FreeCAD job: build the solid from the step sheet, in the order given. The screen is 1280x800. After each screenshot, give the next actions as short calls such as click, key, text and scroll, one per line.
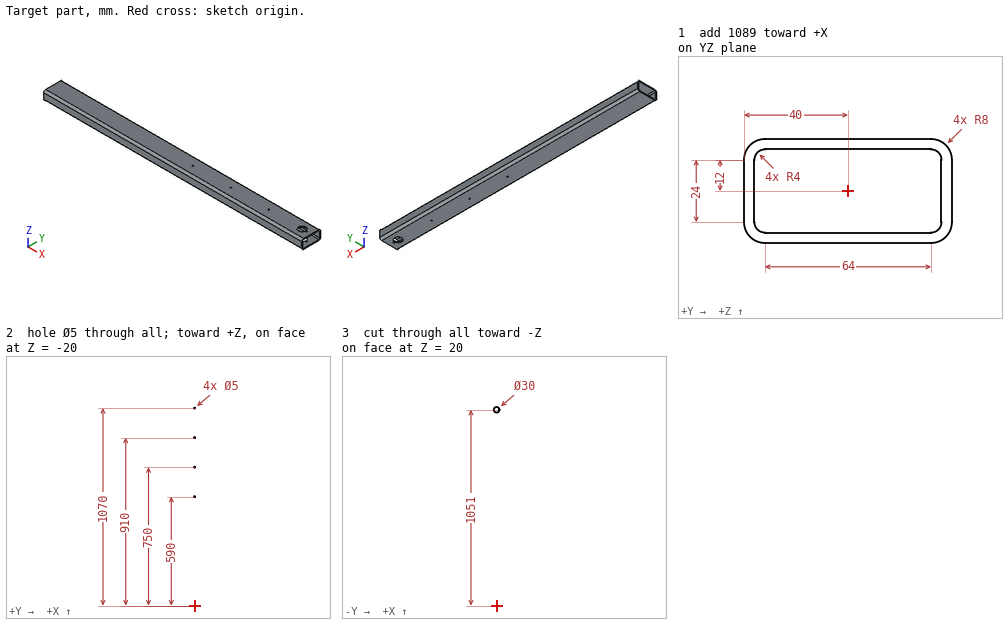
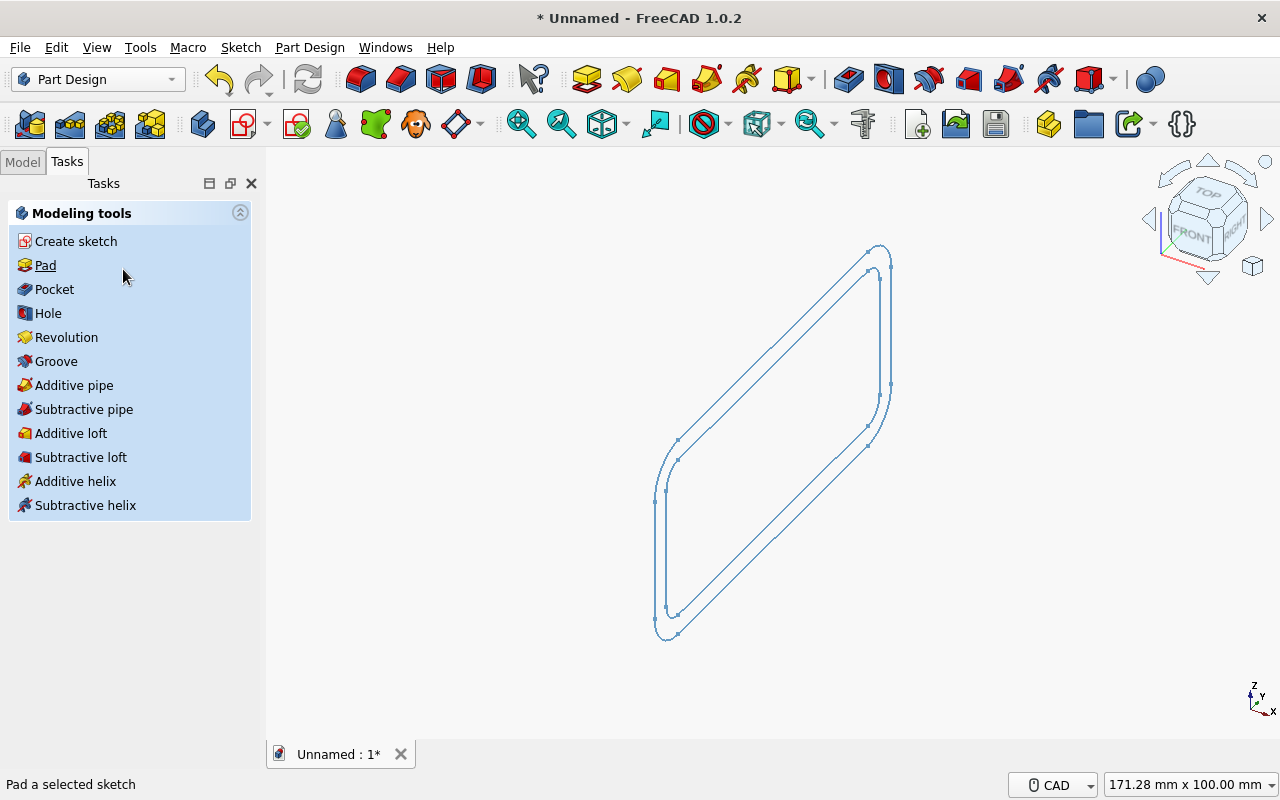
click(588, 80)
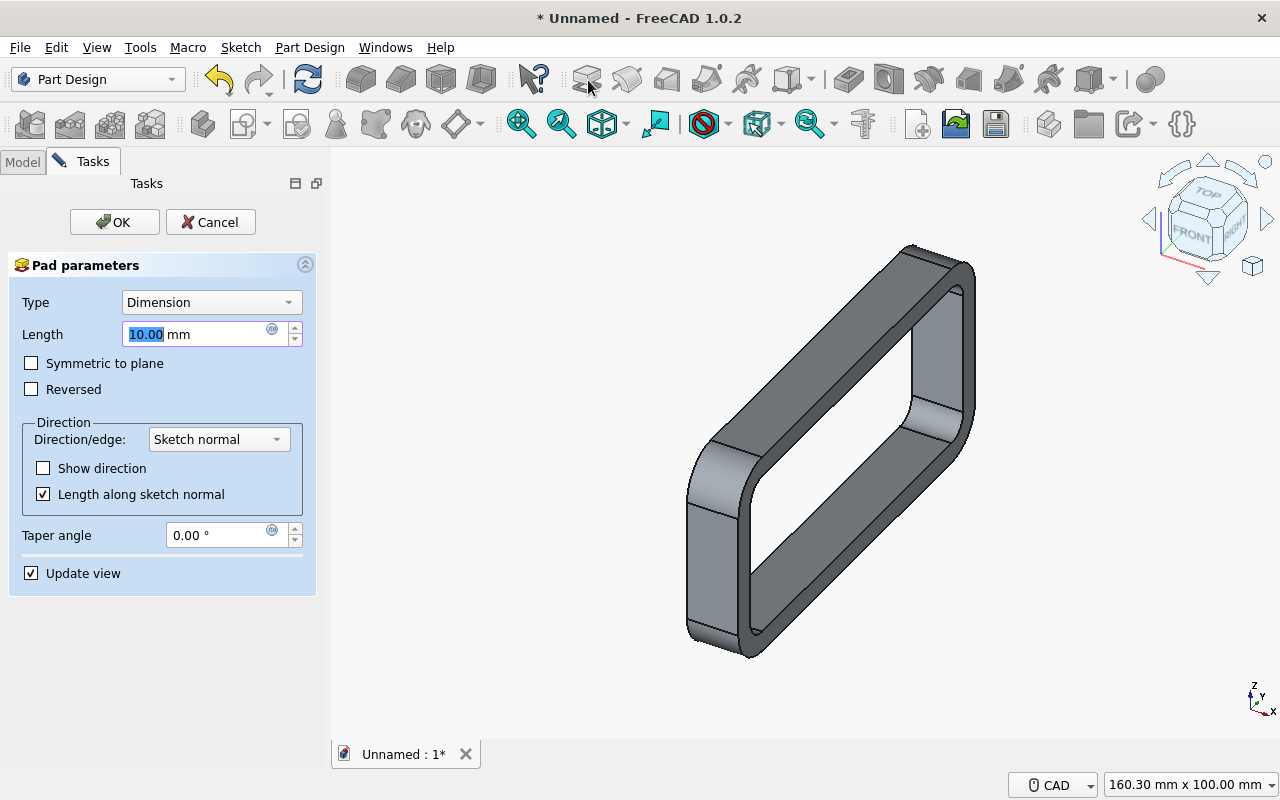
text(1089)
key(Tab)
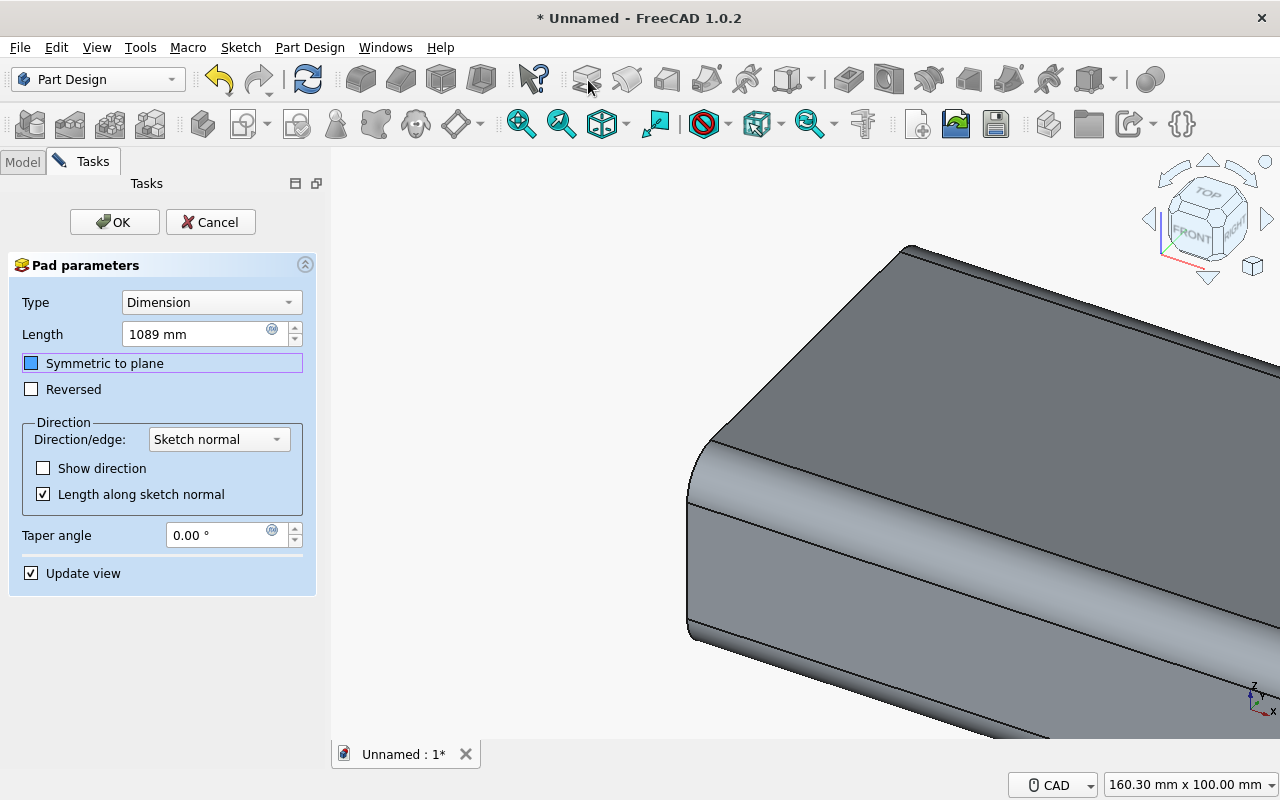
click(115, 222)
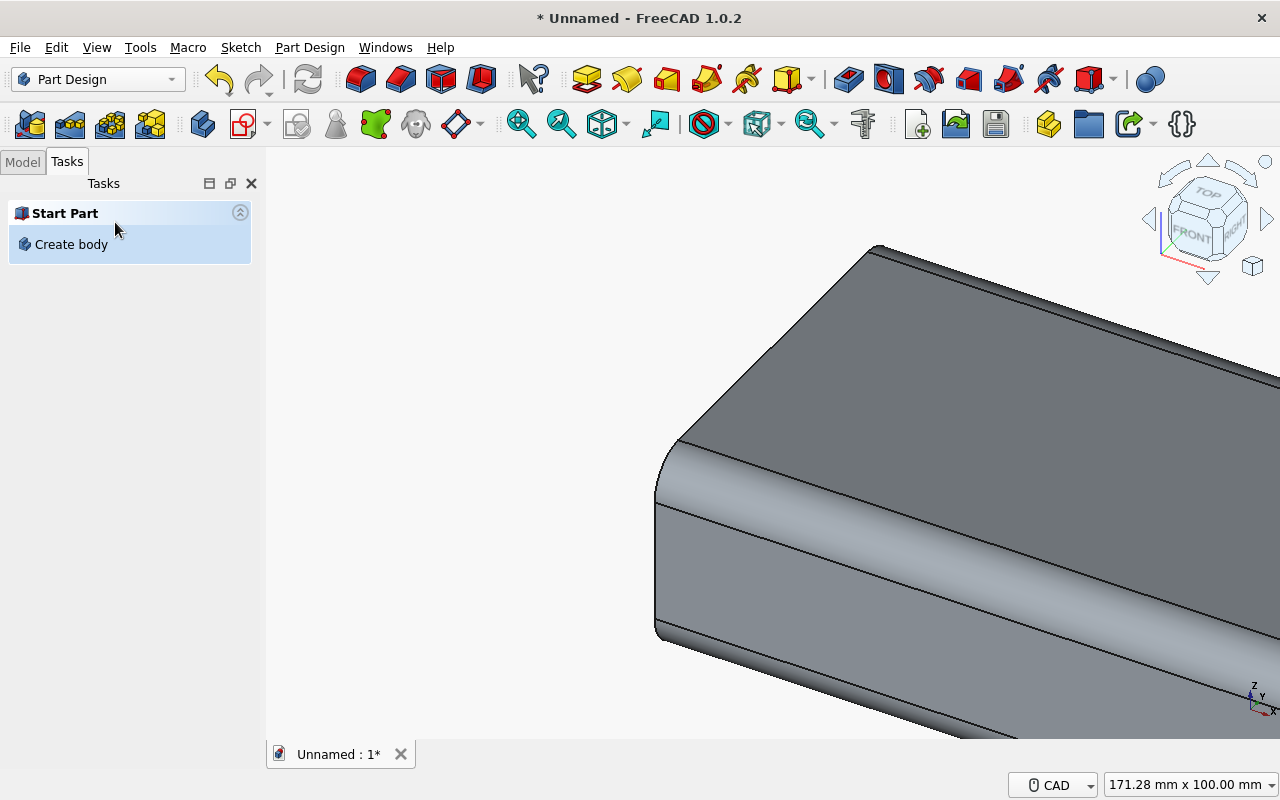
click(522, 124)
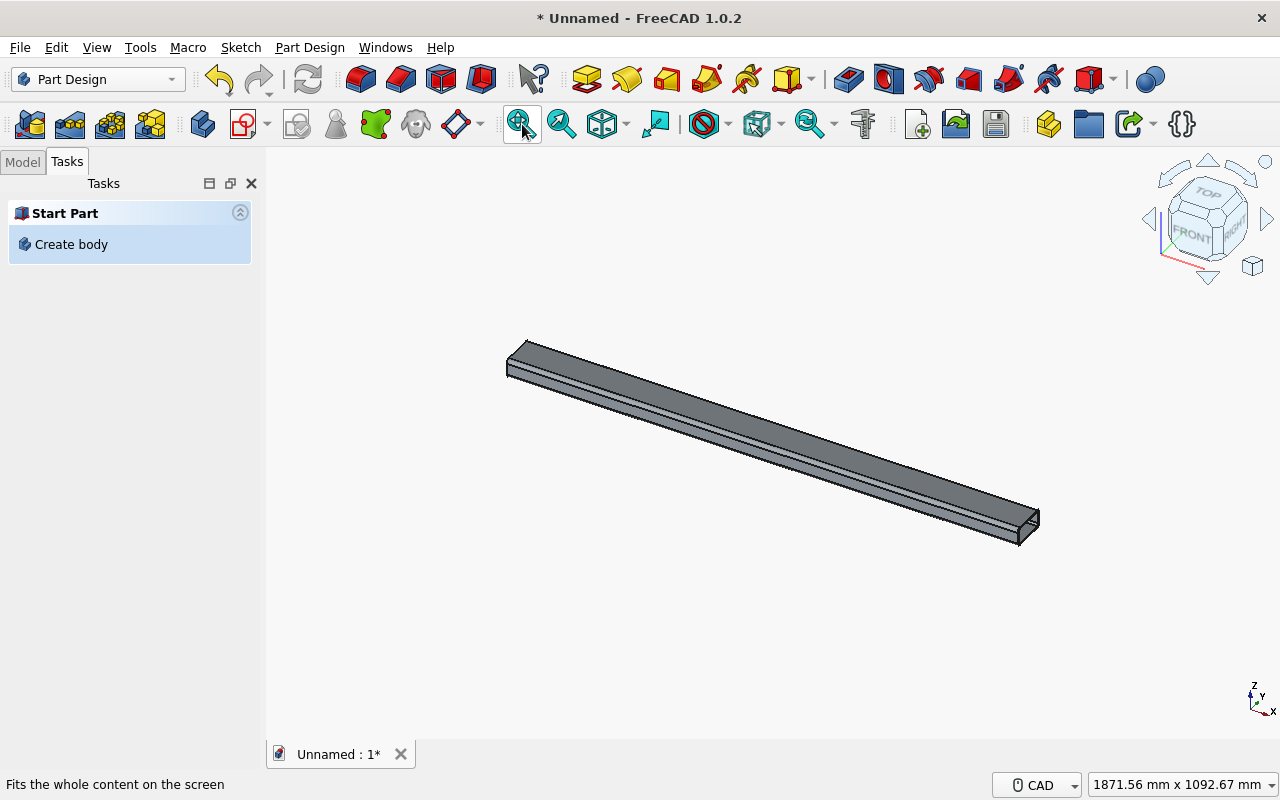
key(5)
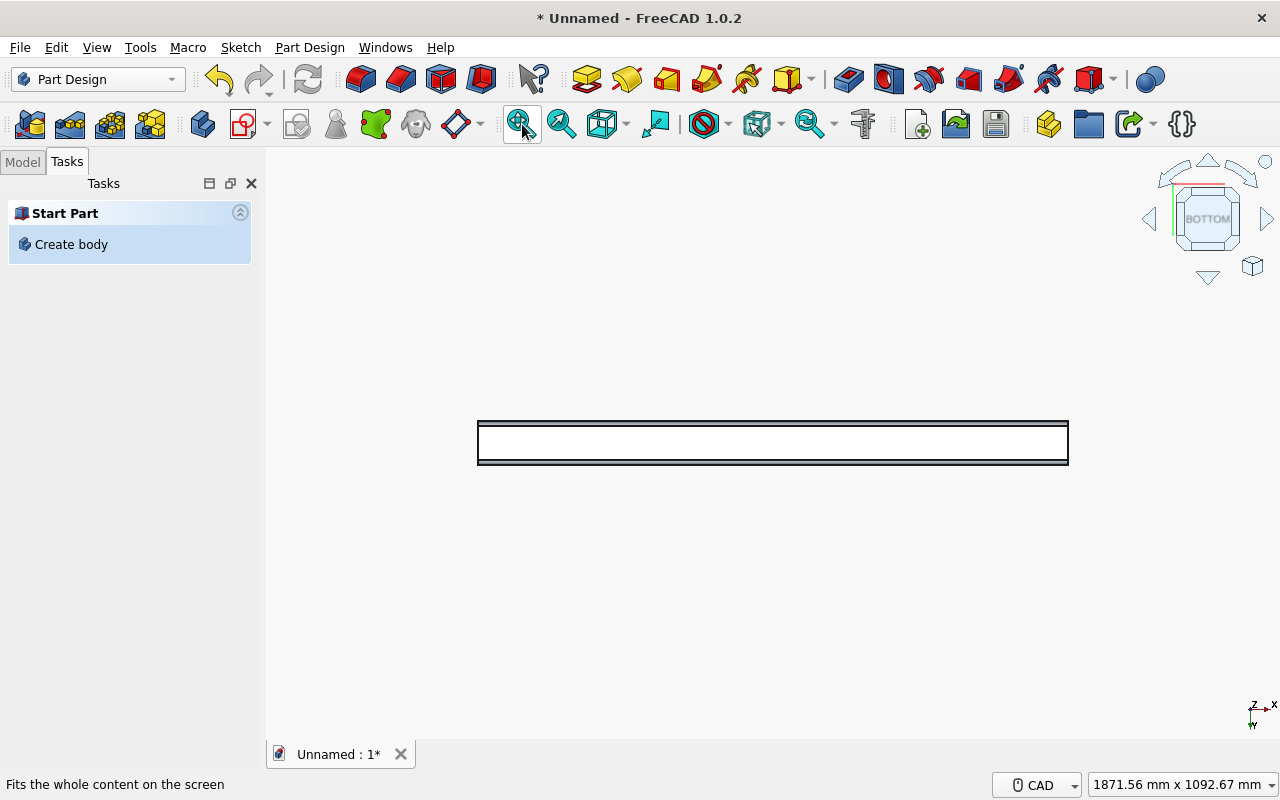
click(773, 442)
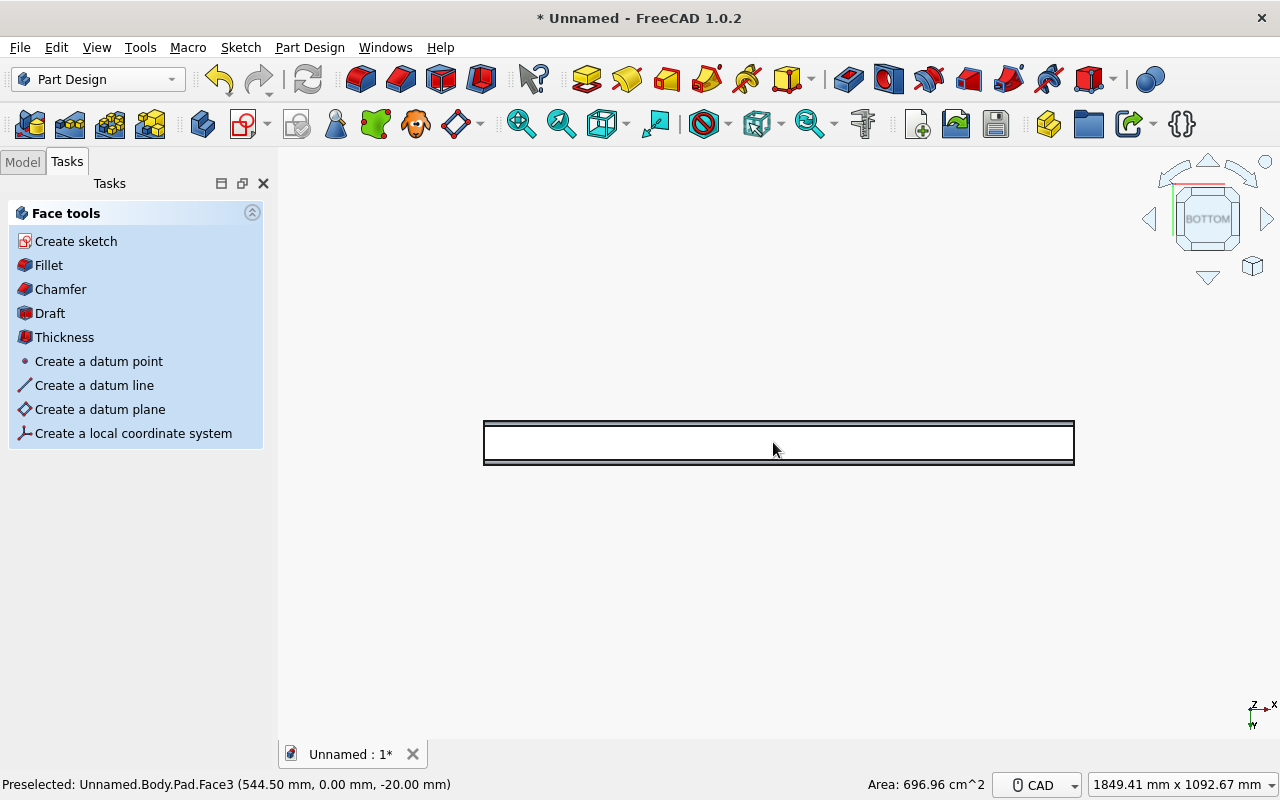
click(244, 124)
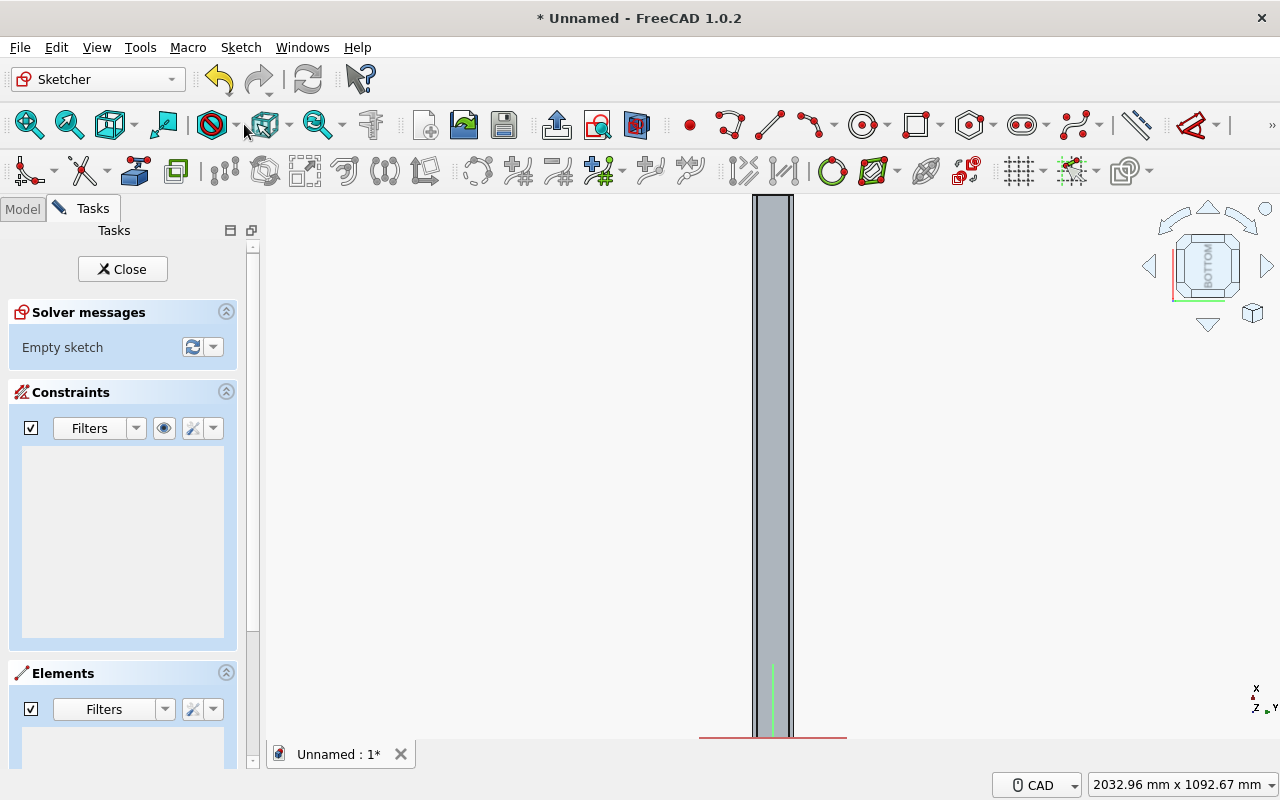
scroll(565, 458, down, 2)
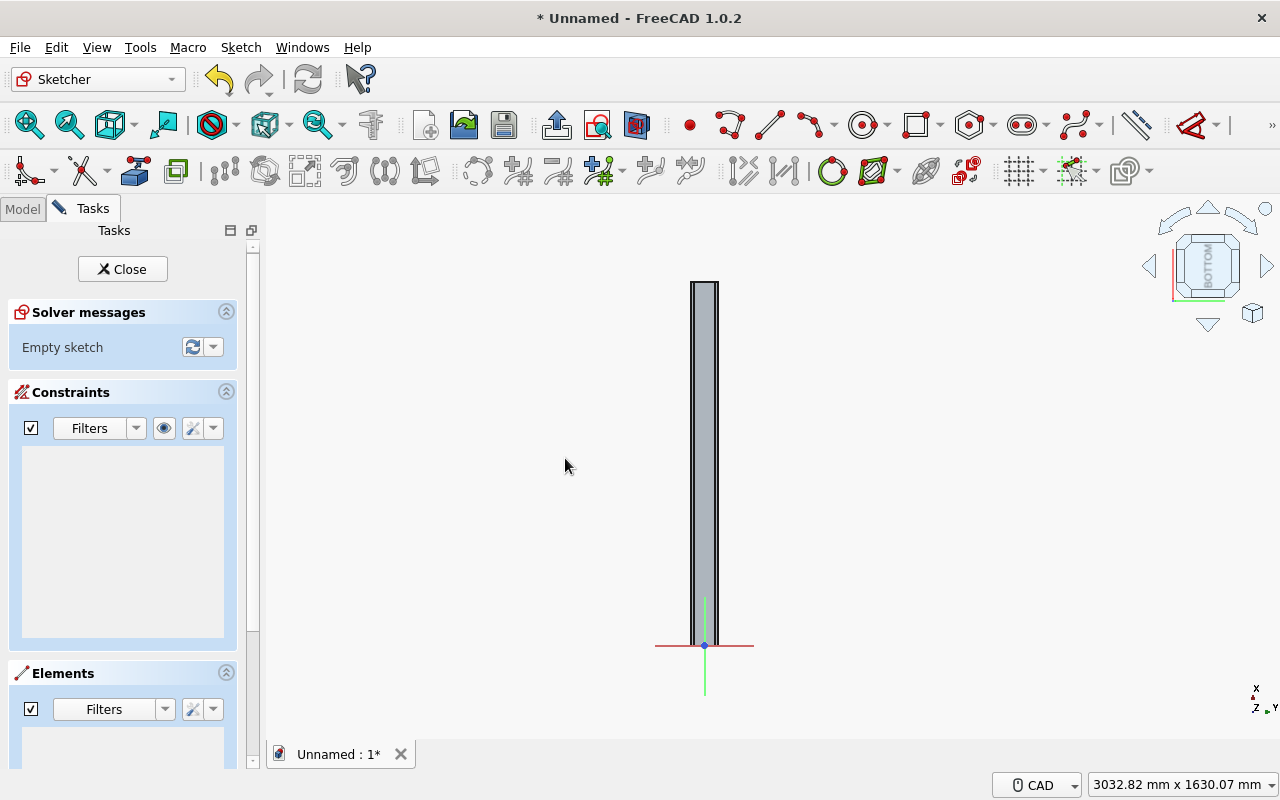
click(864, 126)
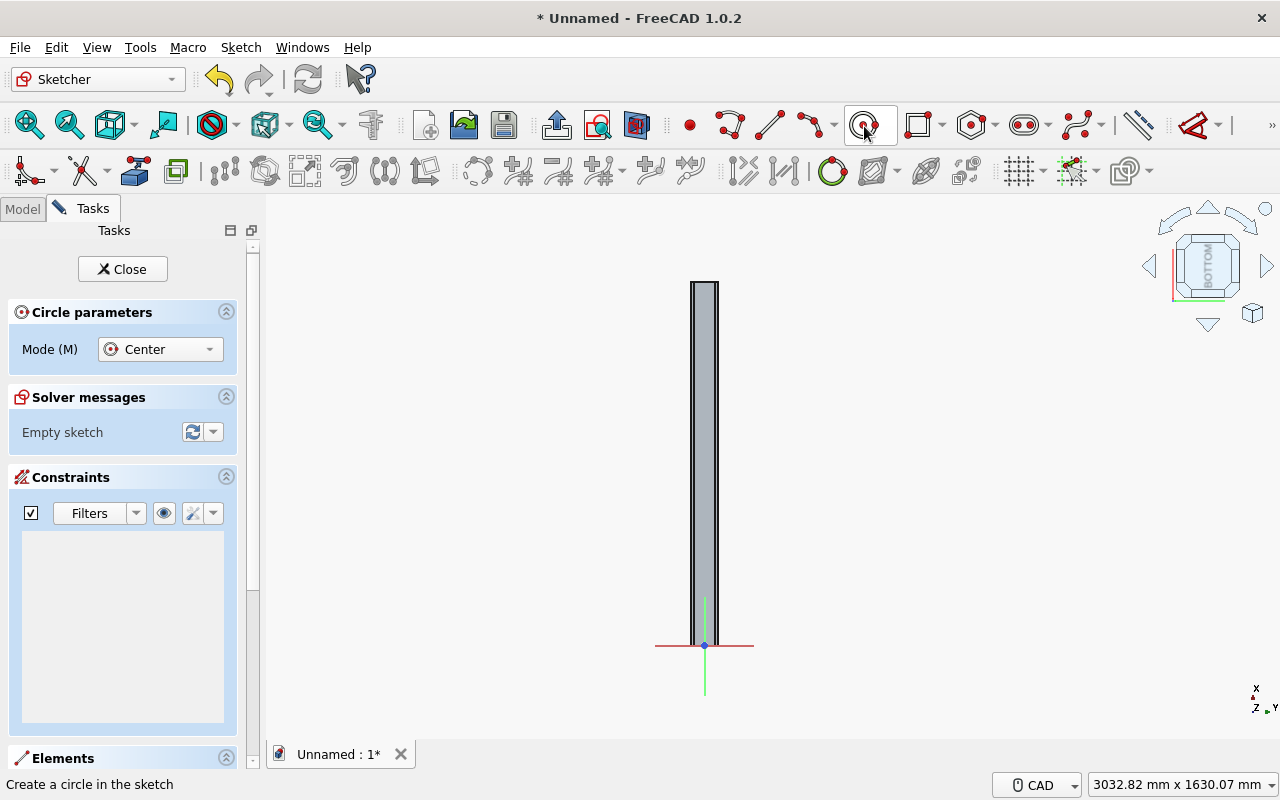
scroll(705, 449, up, 17)